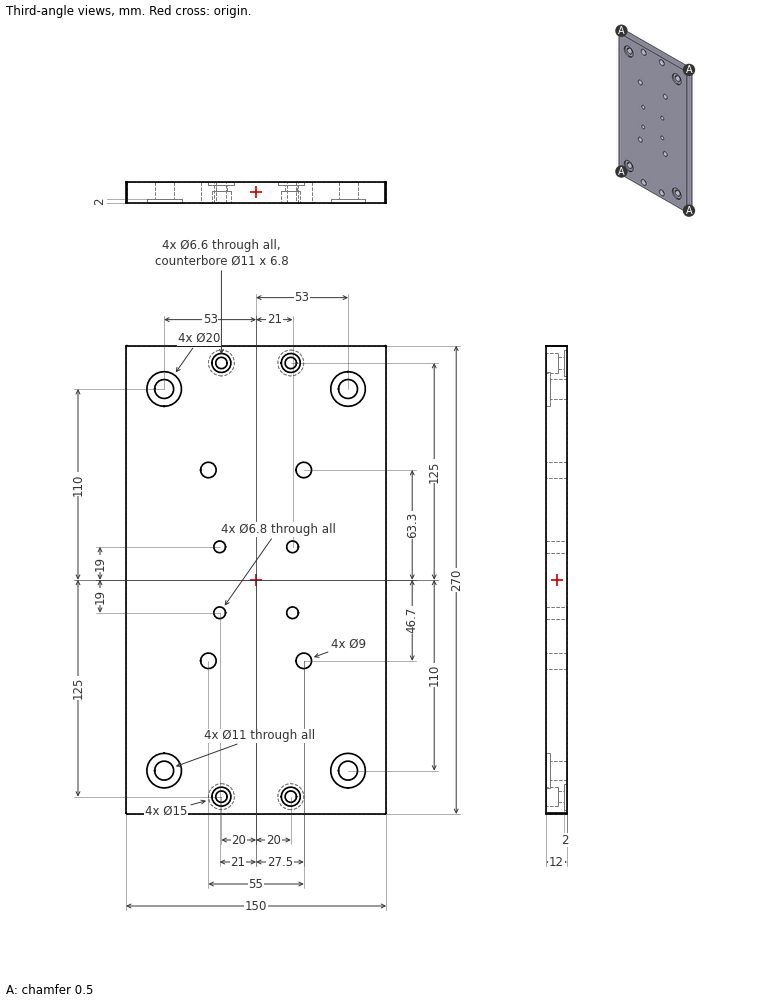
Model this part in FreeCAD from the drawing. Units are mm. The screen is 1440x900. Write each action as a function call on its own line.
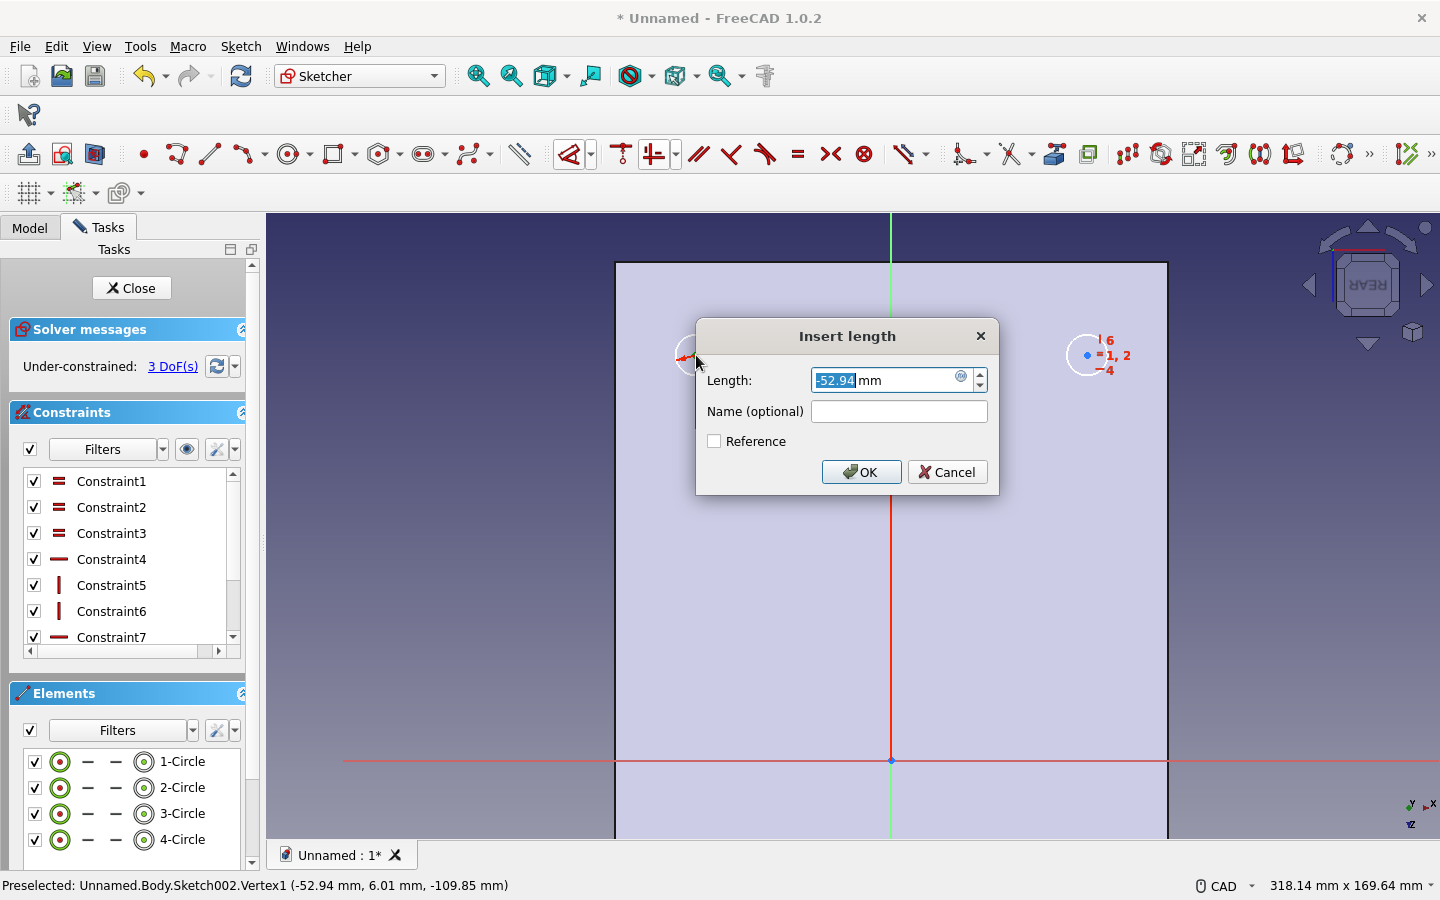
text(-53)
key(Return)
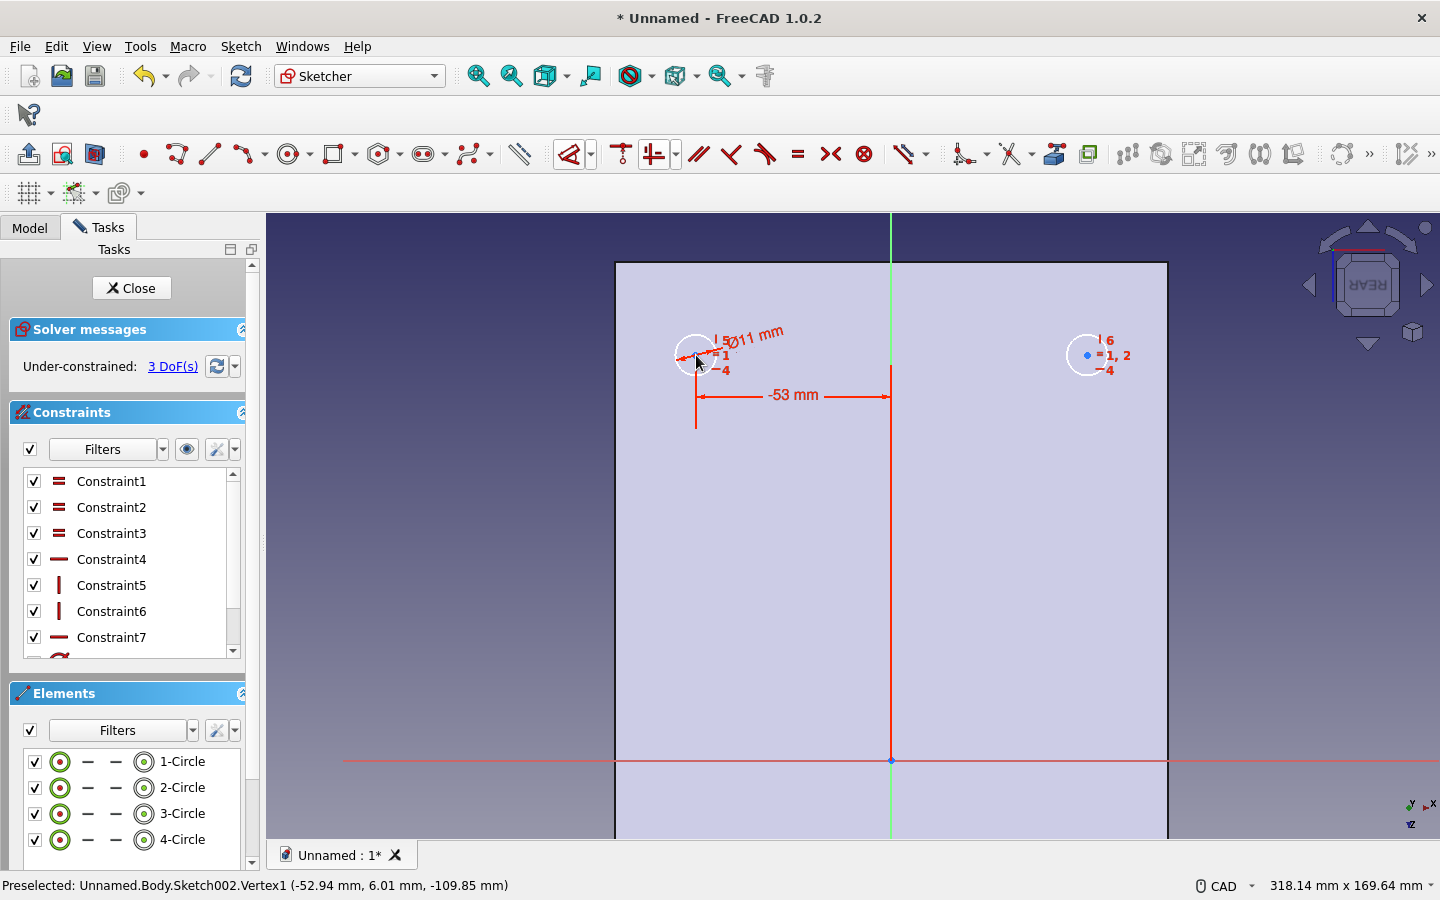
click(1087, 355)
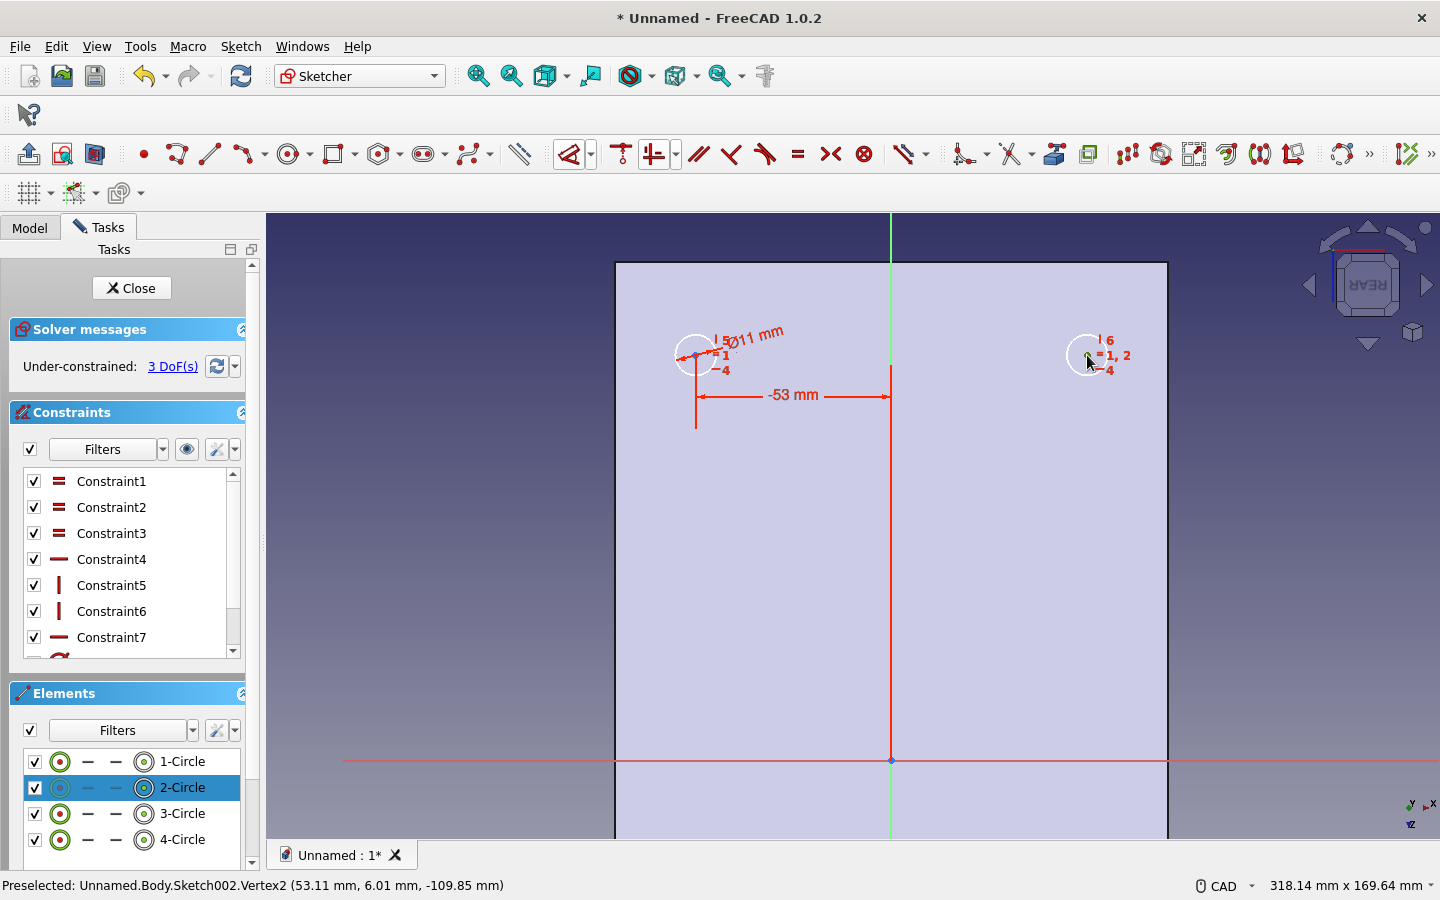
click(590, 154)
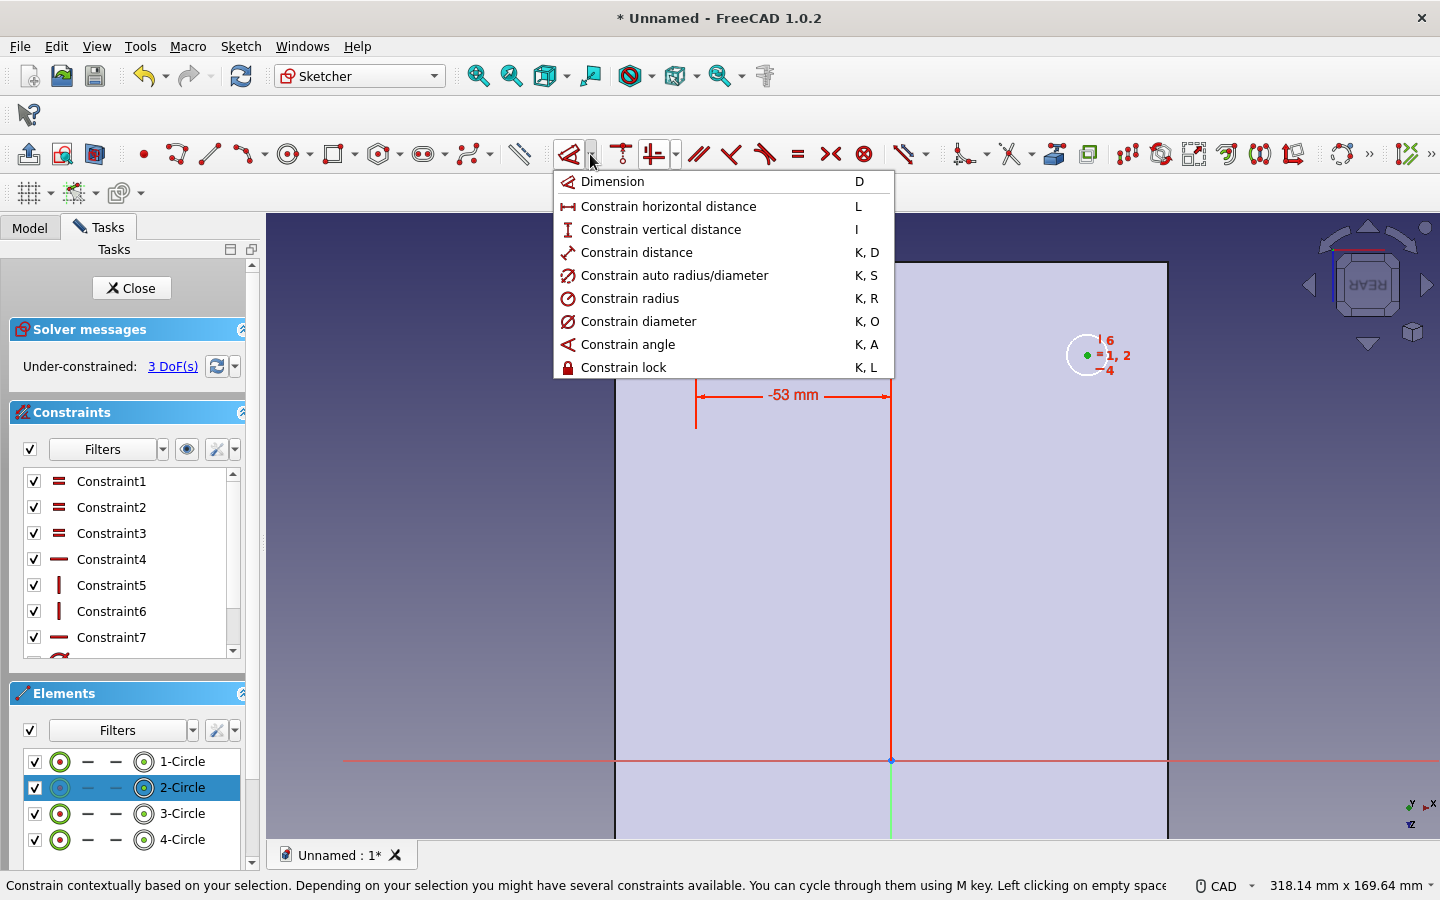
click(724, 206)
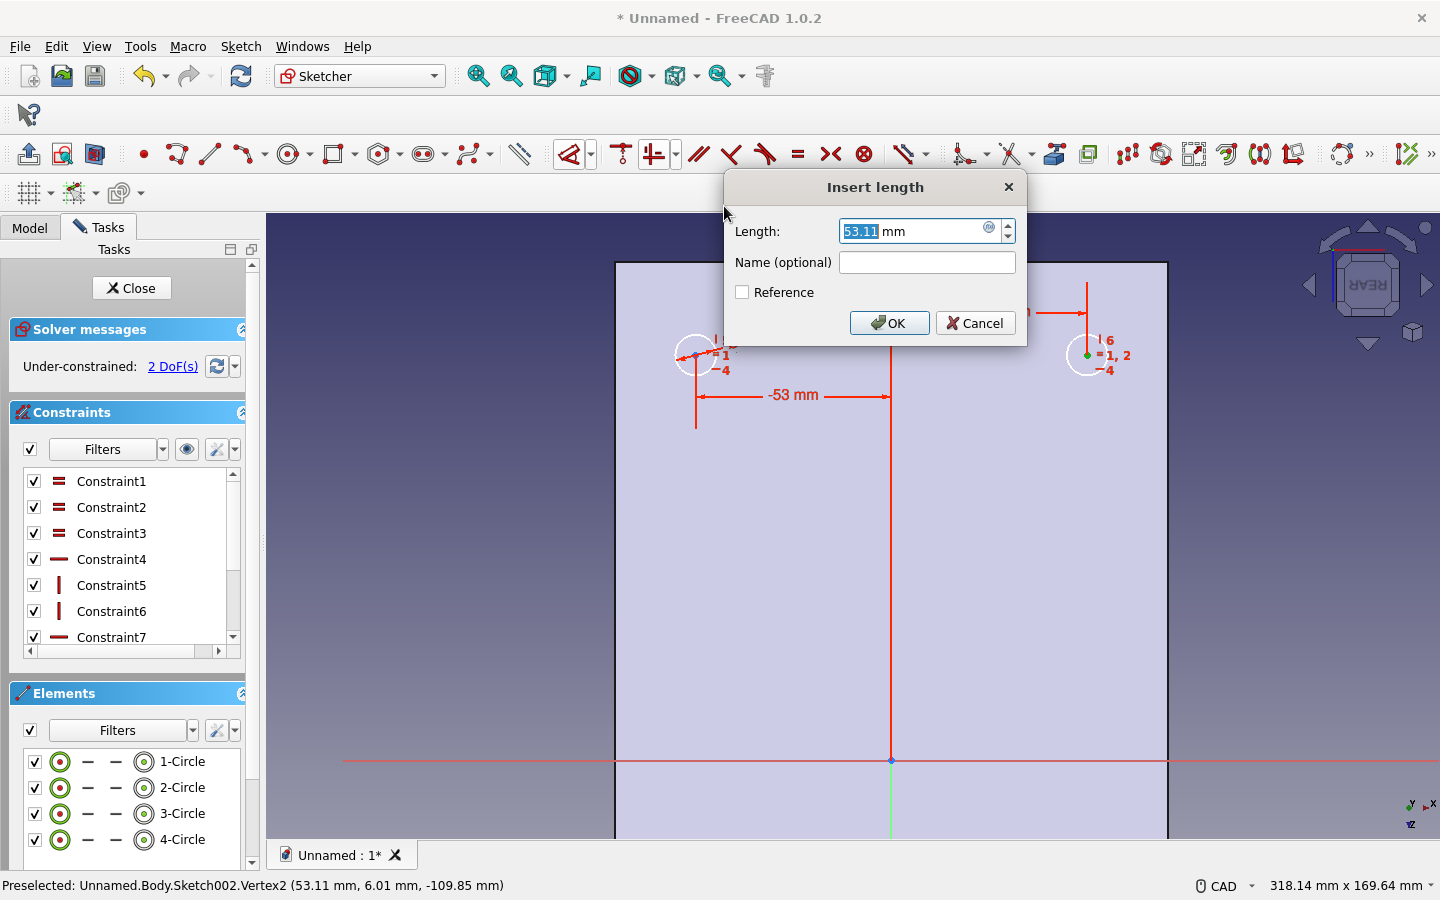
text(53)
key(Return)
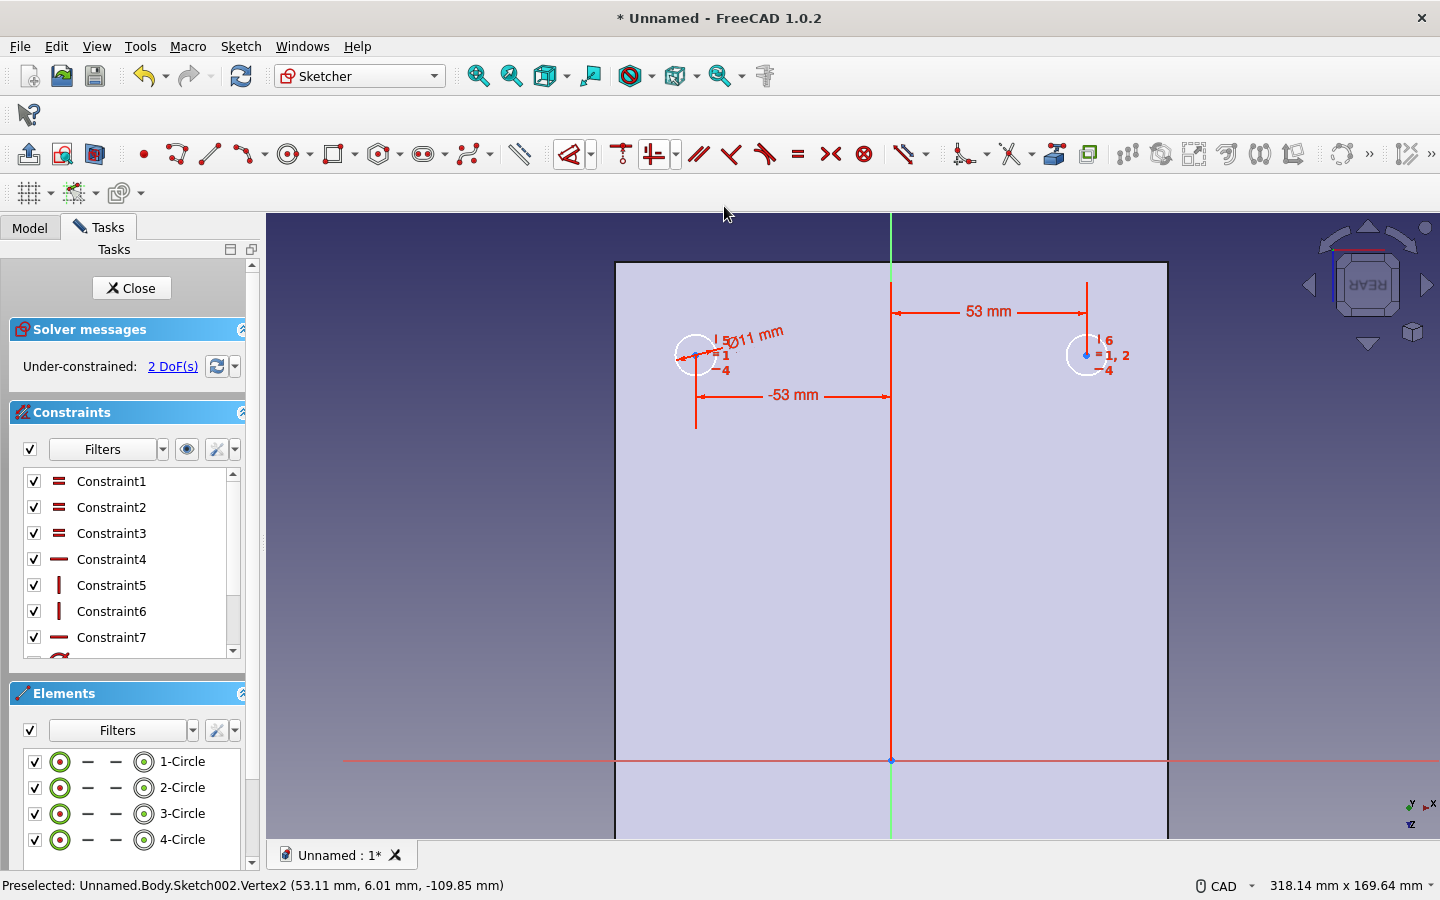
click(696, 355)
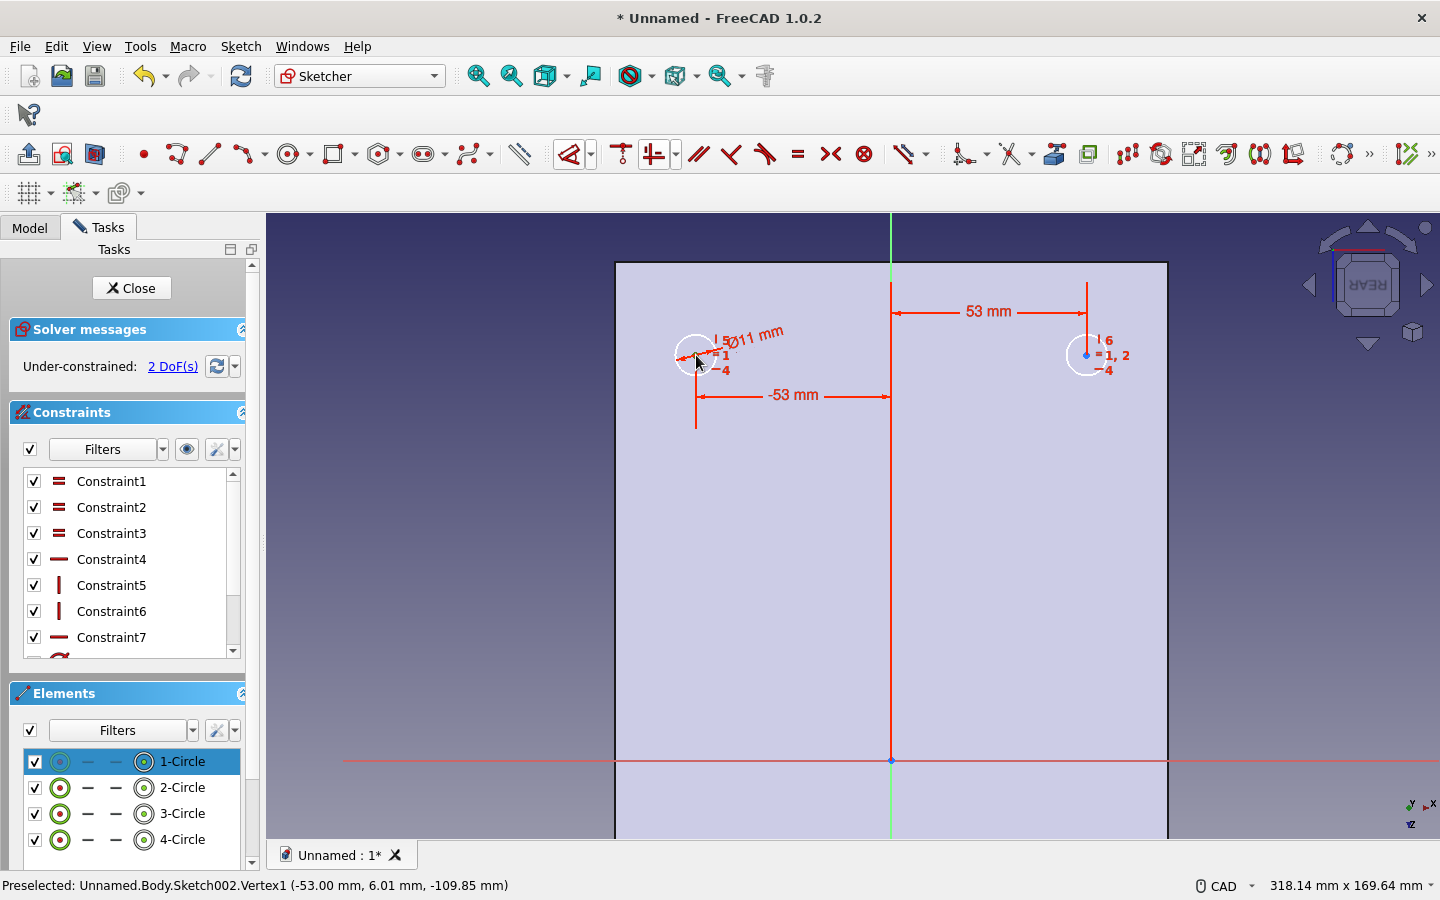
key(i)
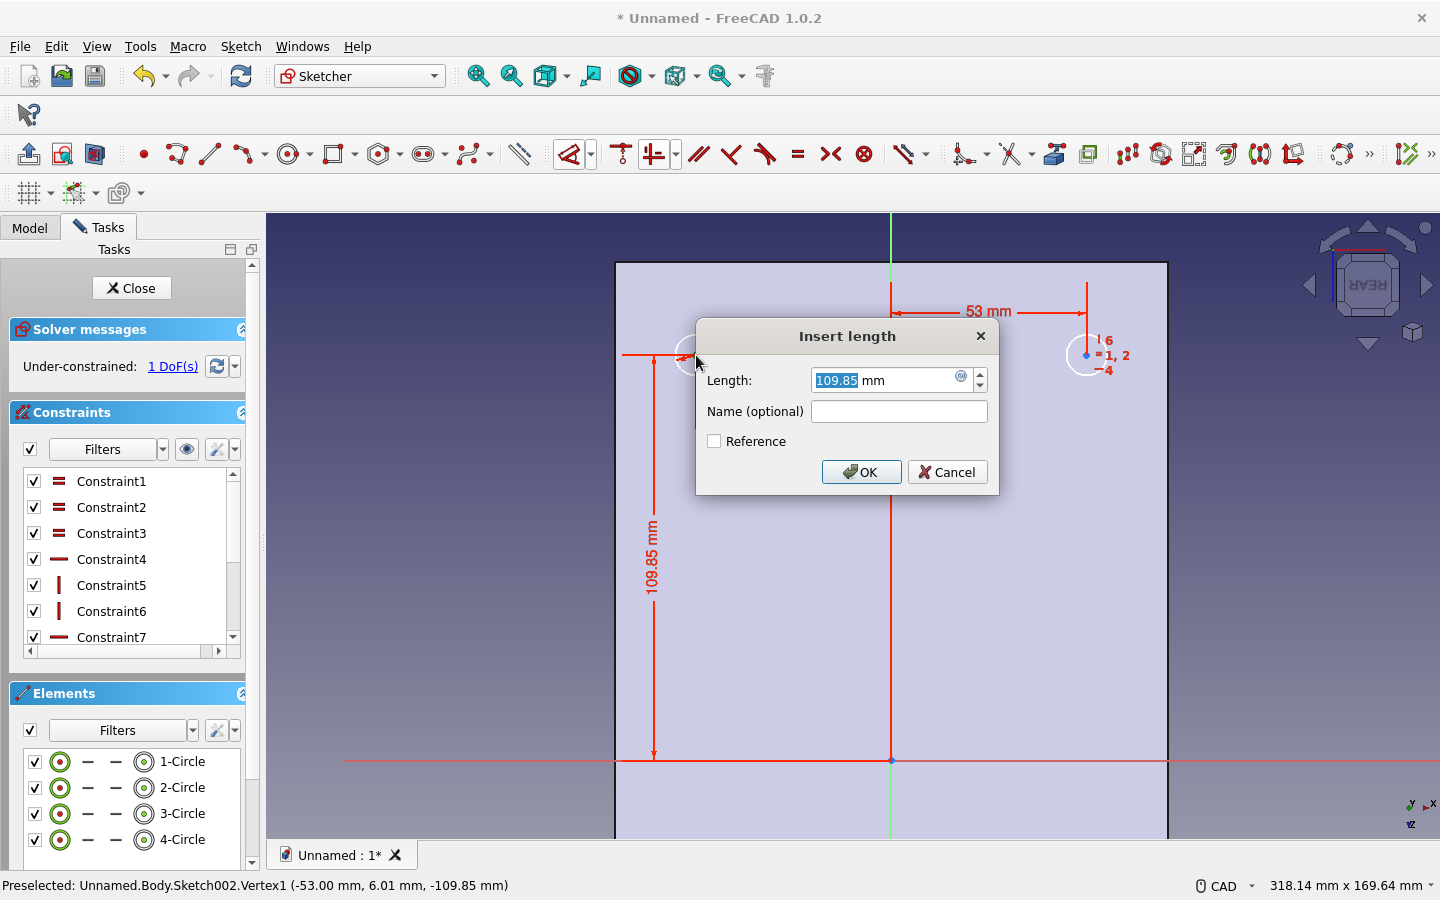
text(110)
key(Return)